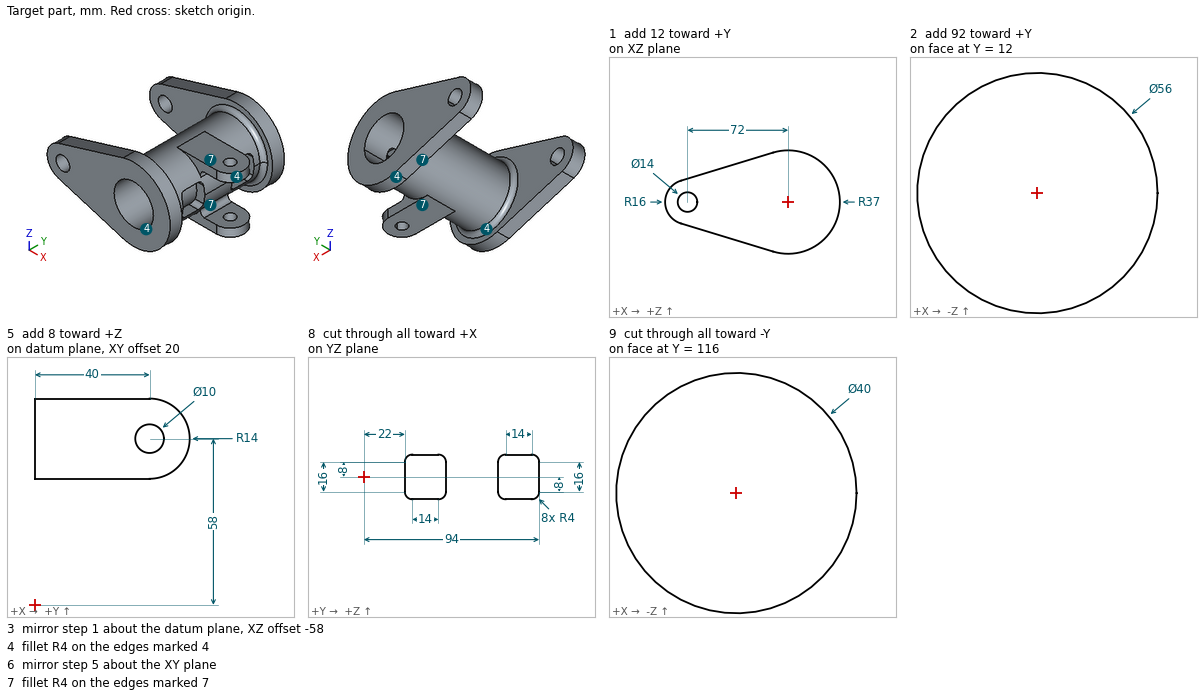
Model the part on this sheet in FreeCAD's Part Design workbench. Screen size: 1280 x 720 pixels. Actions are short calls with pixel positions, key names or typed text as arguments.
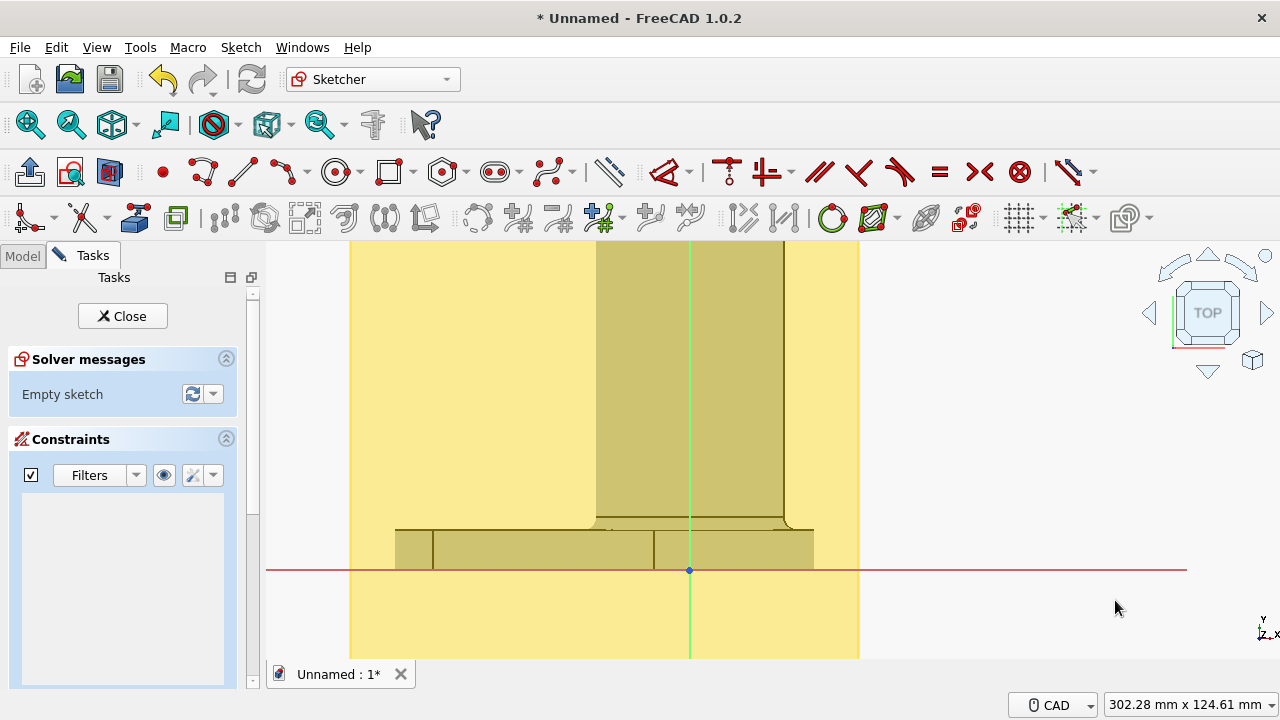
click(204, 172)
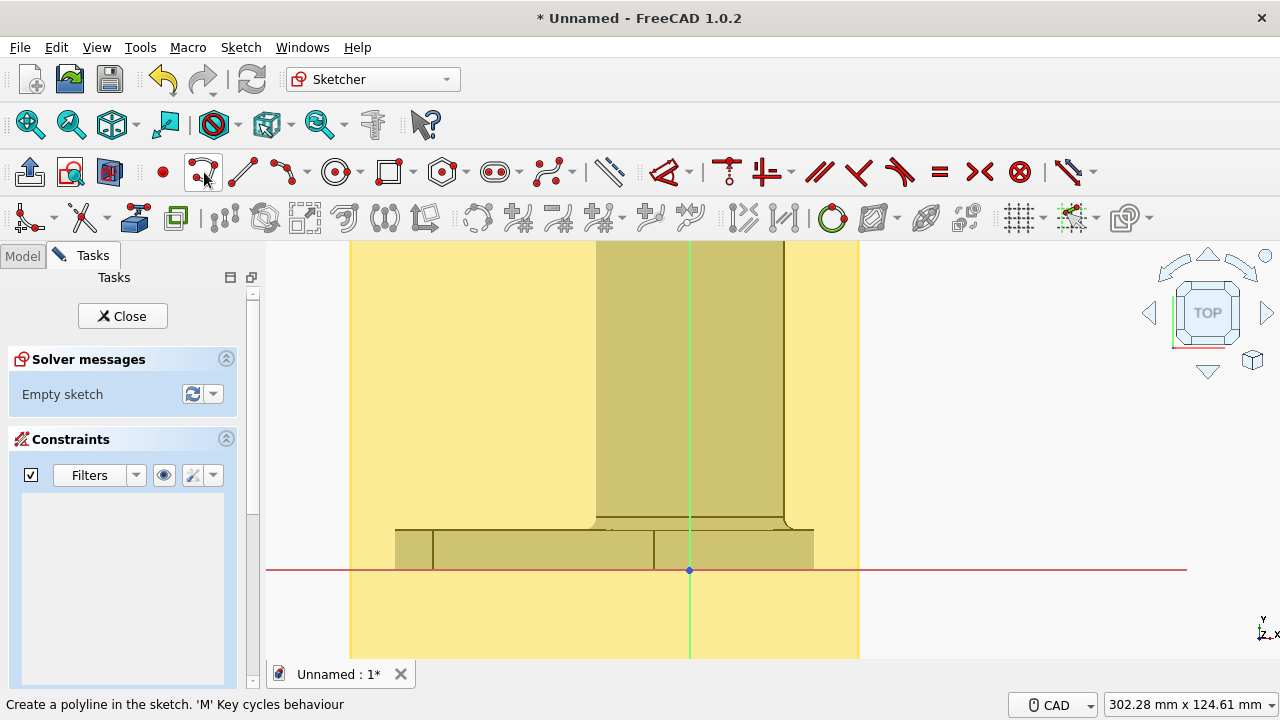
click(824, 329)
click(690, 329)
click(699, 423)
click(824, 423)
right_click(824, 423)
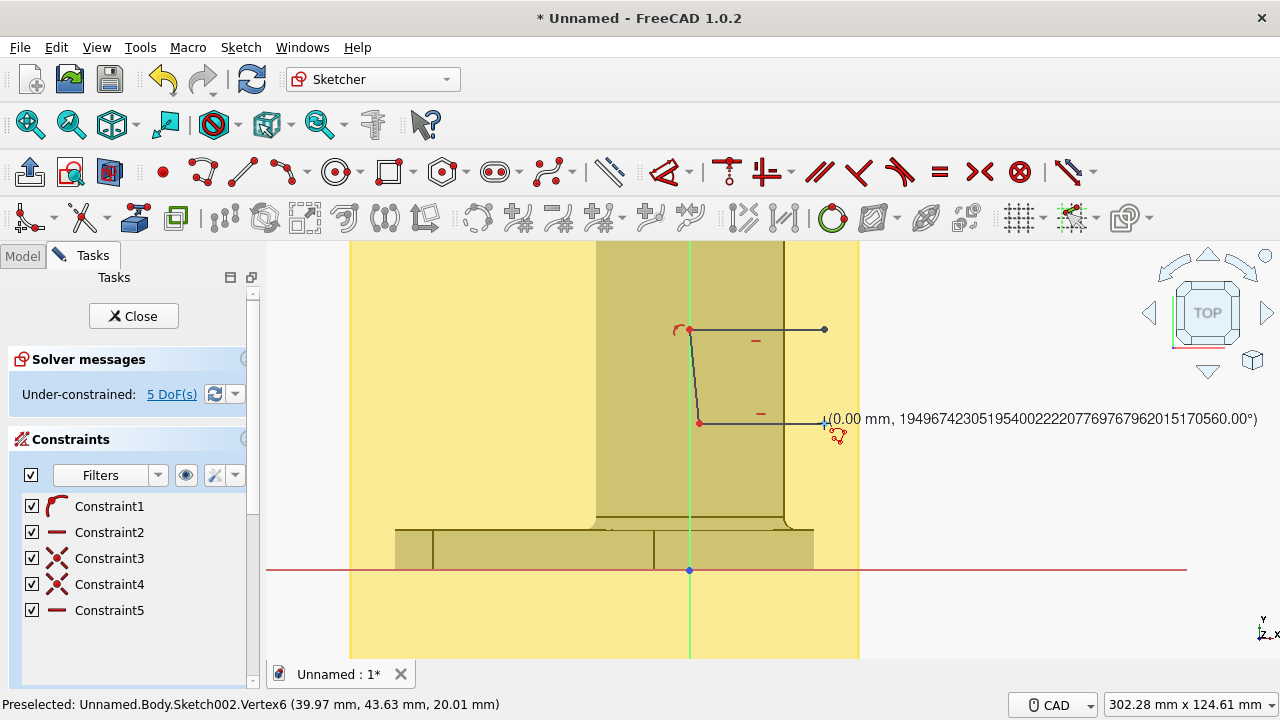
key(g)
key(3)
key(a)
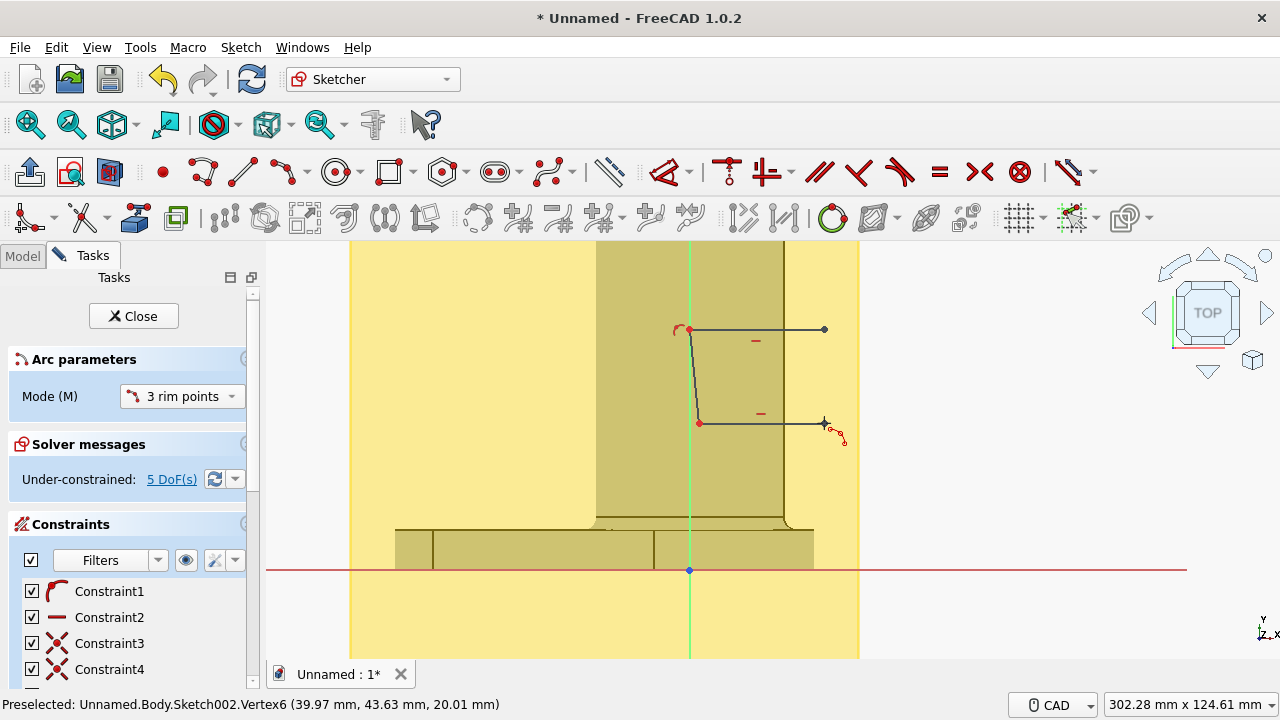
click(824, 424)
click(824, 330)
click(871, 376)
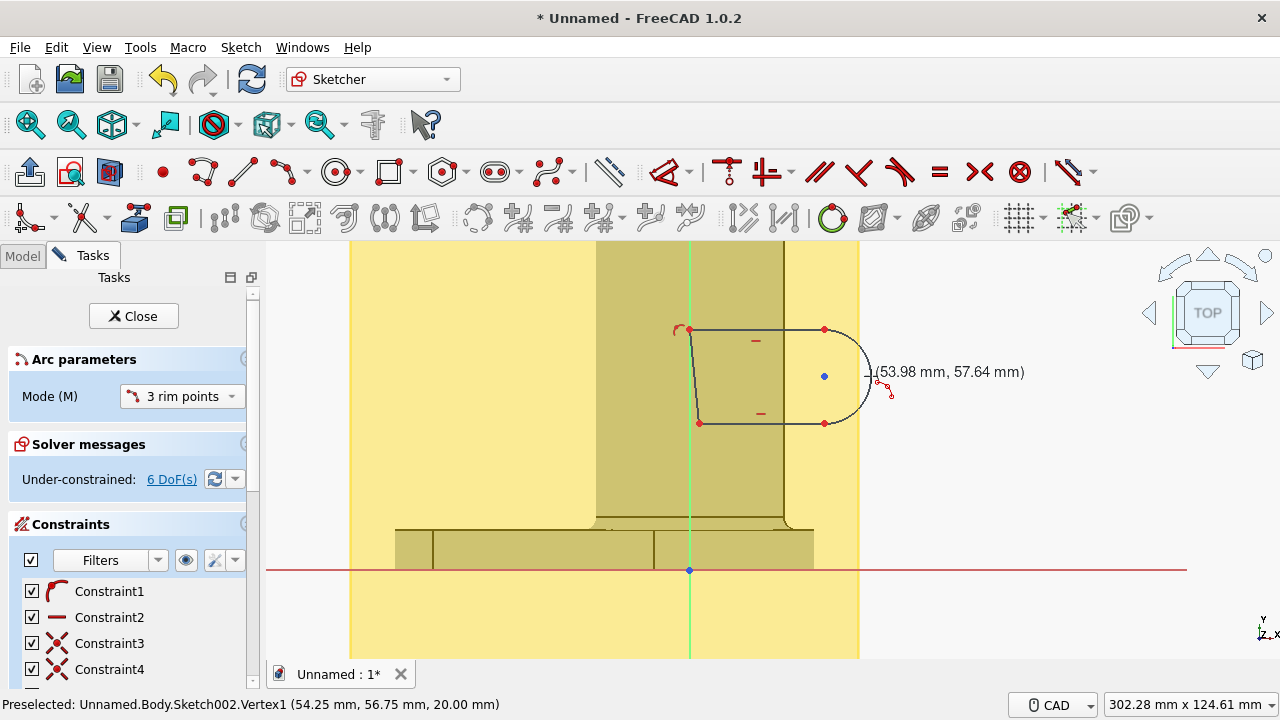
click(336, 172)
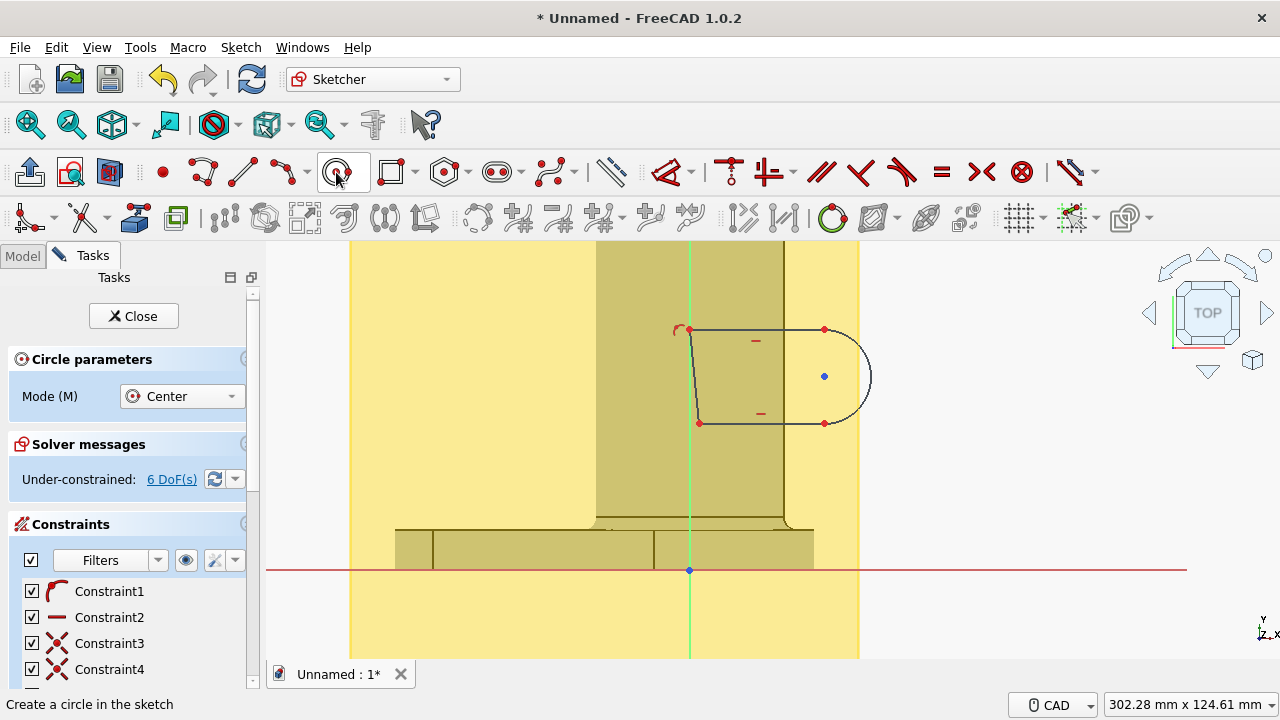
scroll(824, 376, up, 2)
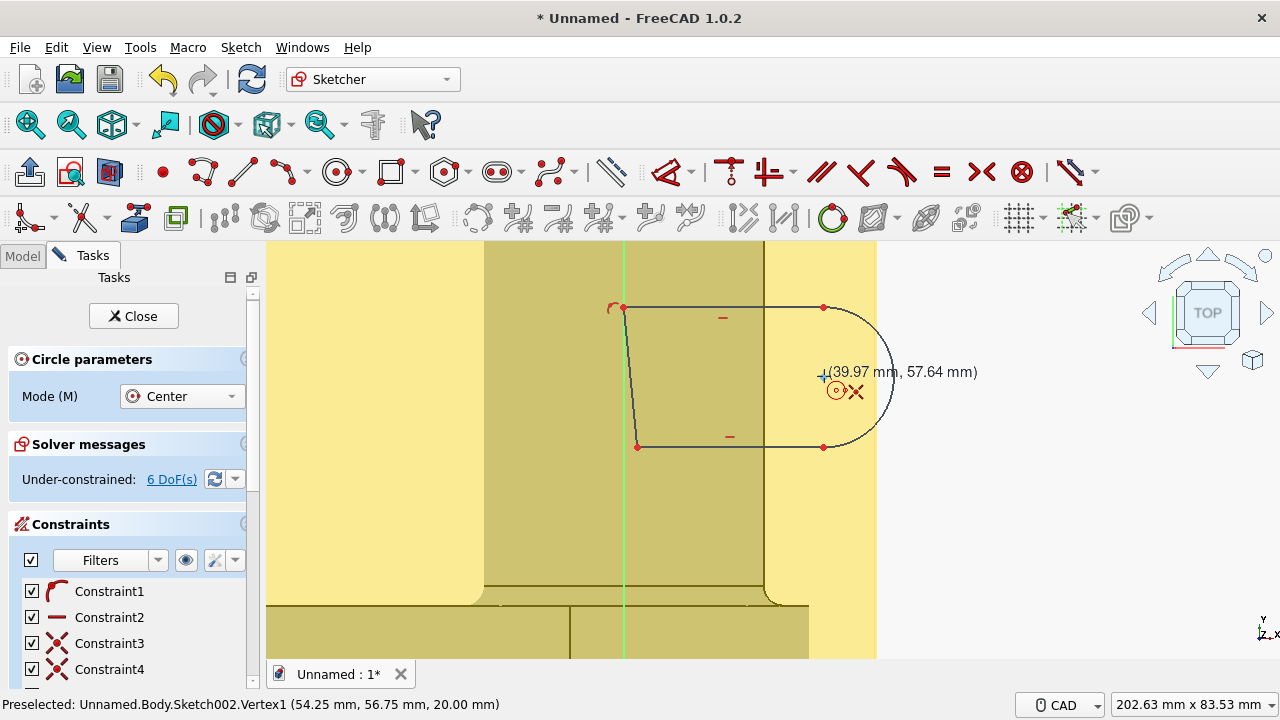
click(824, 376)
move(842, 358)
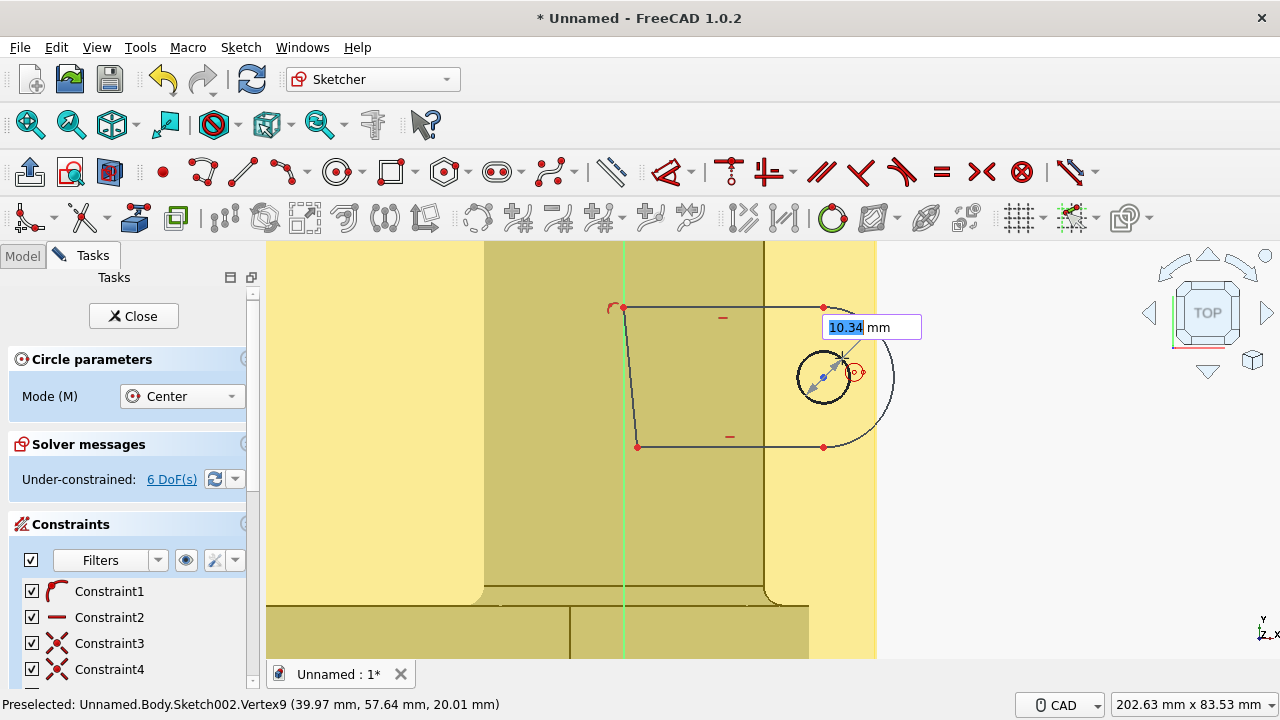
text(10)
key(Return)
key(Escape)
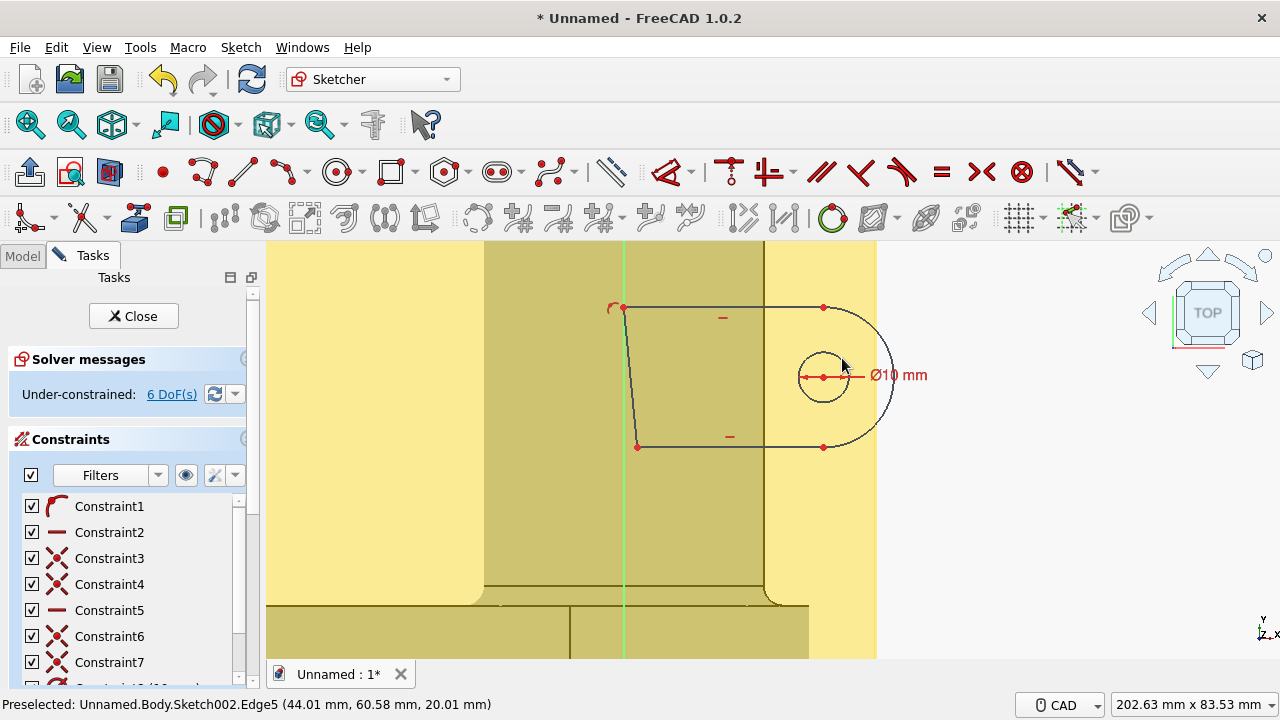
click(764, 307)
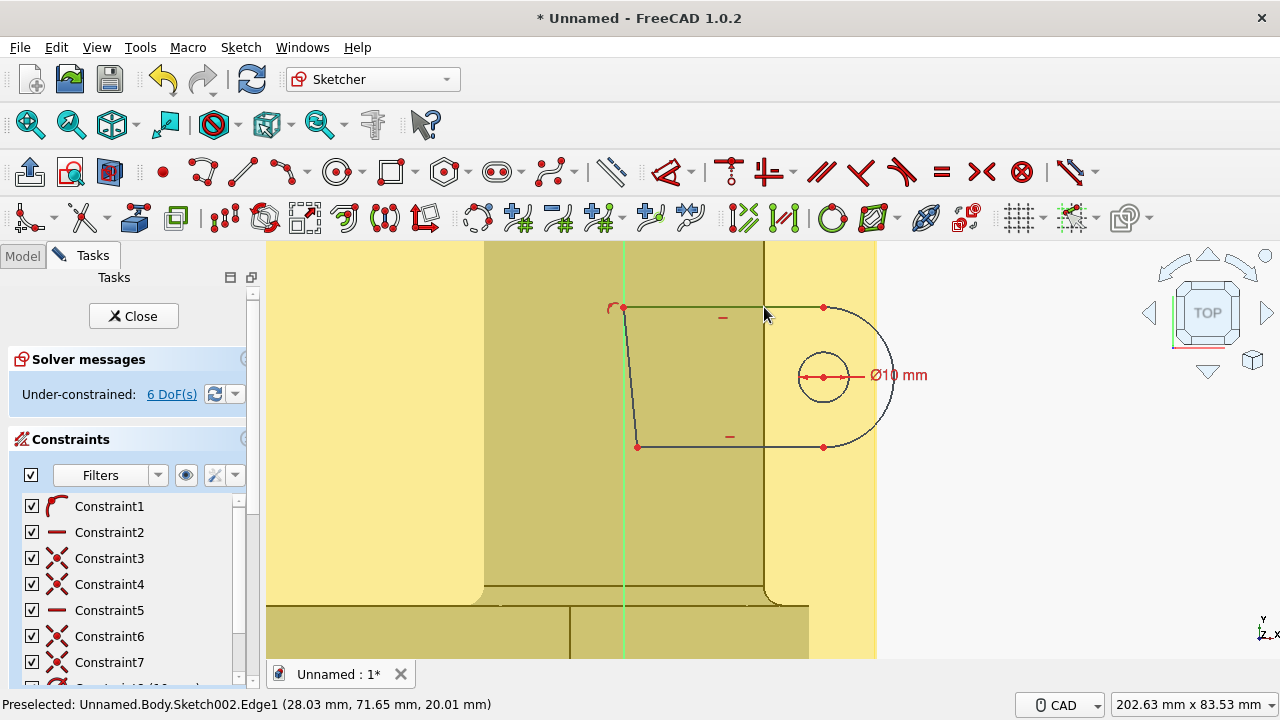
click(880, 419)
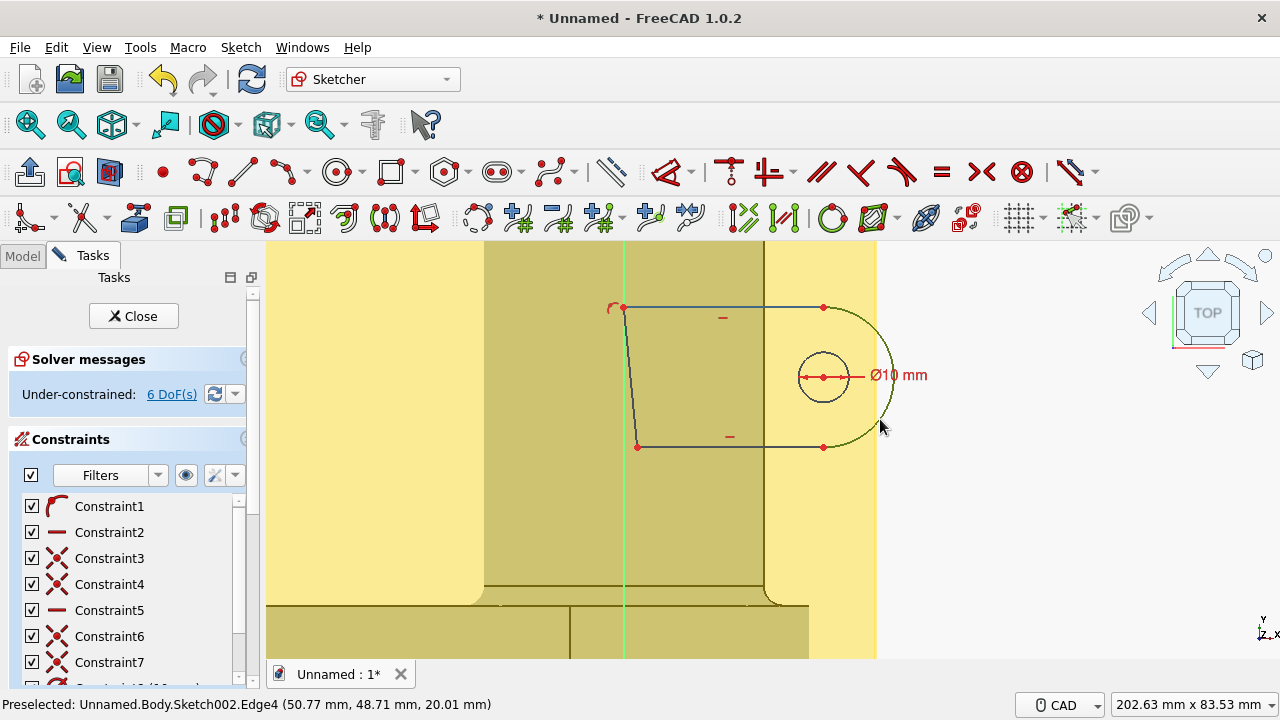
key(t)